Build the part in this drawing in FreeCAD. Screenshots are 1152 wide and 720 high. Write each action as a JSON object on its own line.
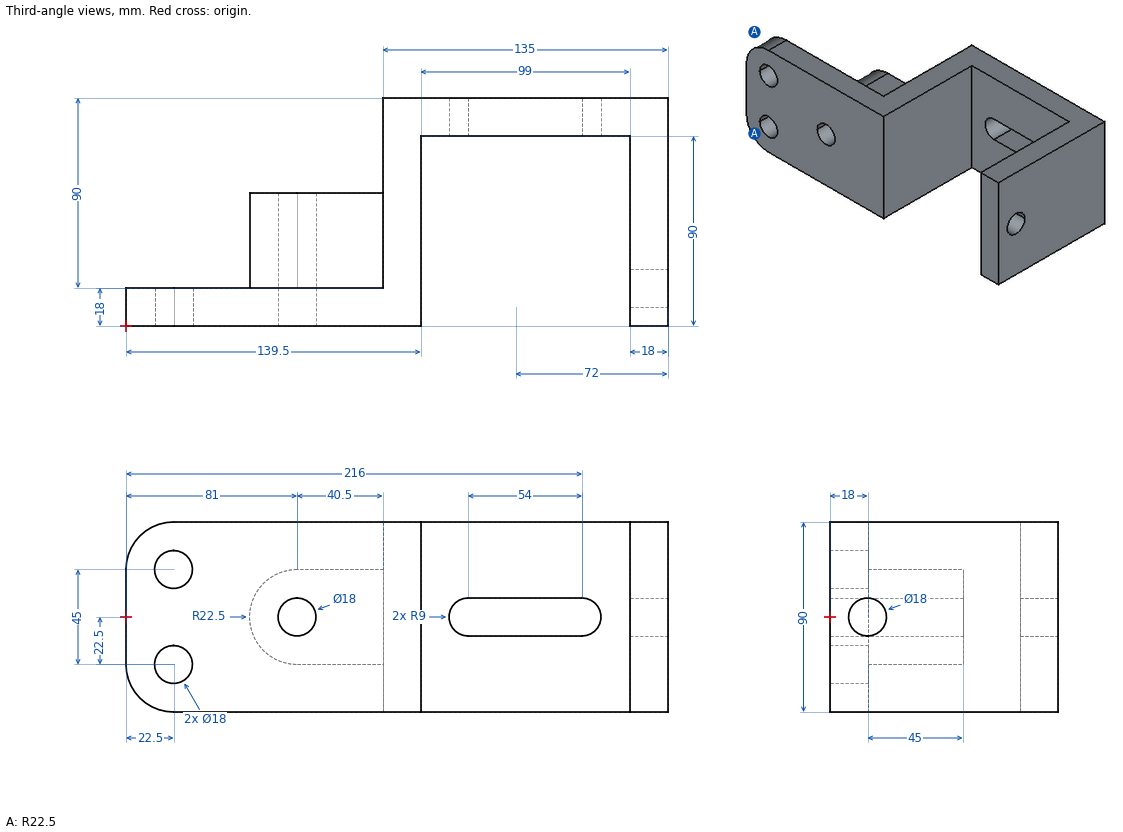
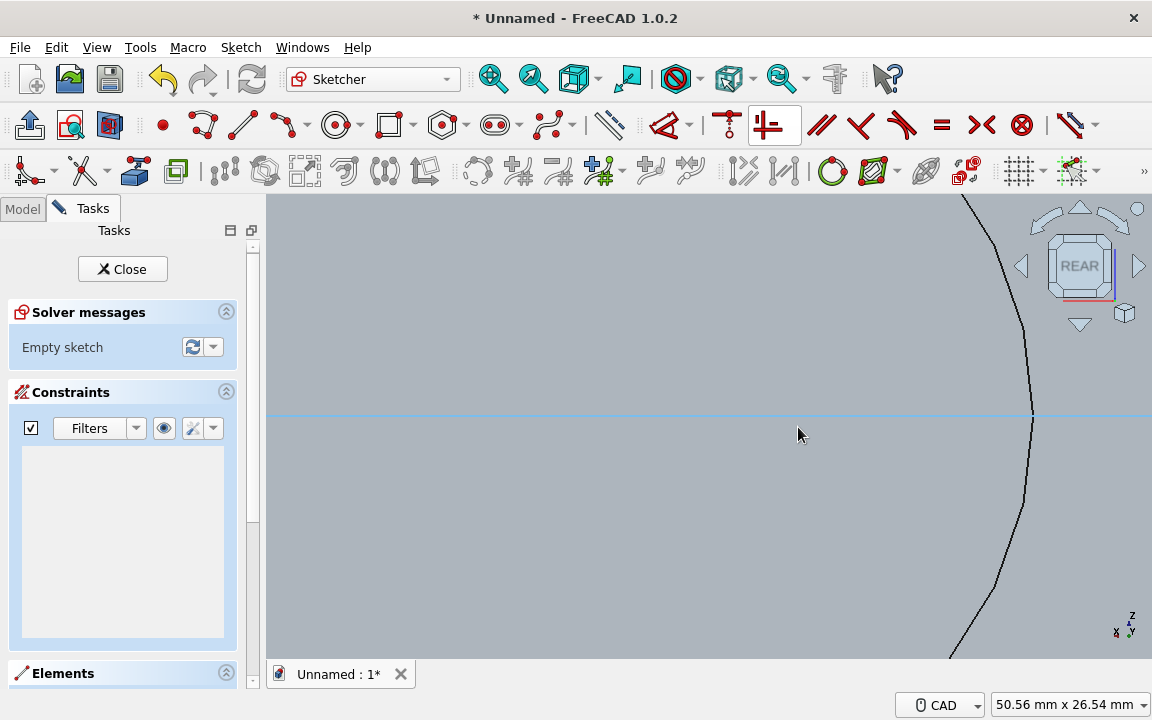
{"action": "left_click", "coordinate": [336, 126]}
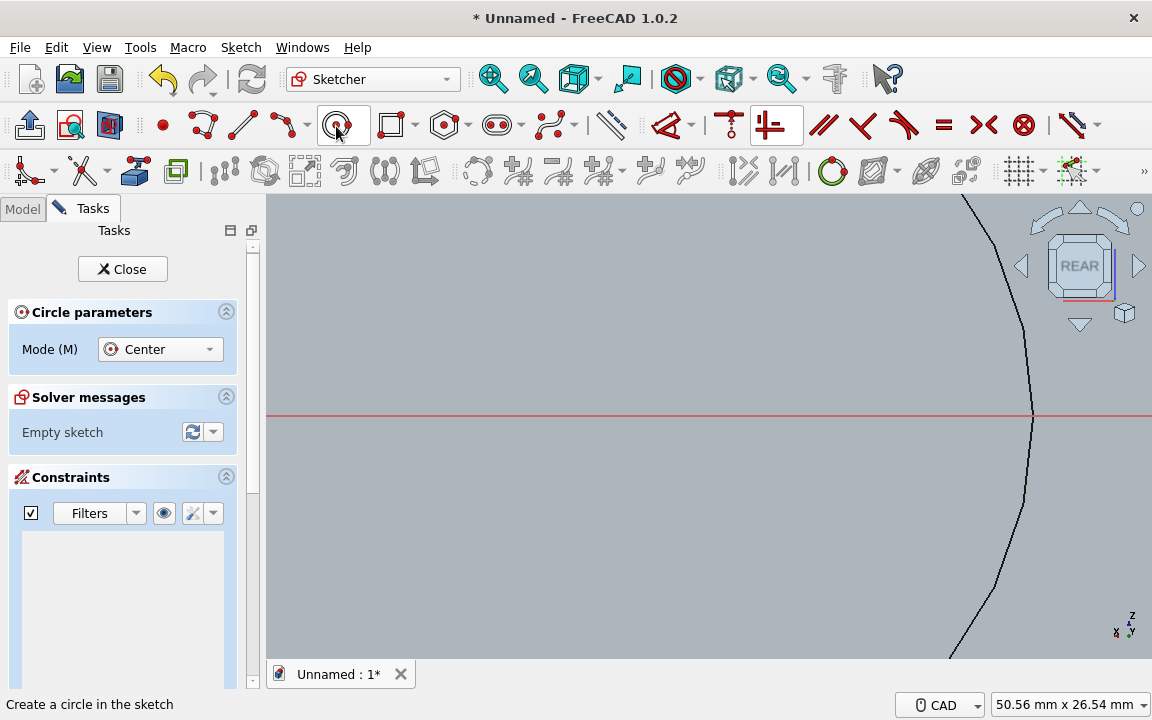
{"action": "left_click", "coordinate": [639, 416]}
{"action": "mouse_move", "coordinate": [750, 305]}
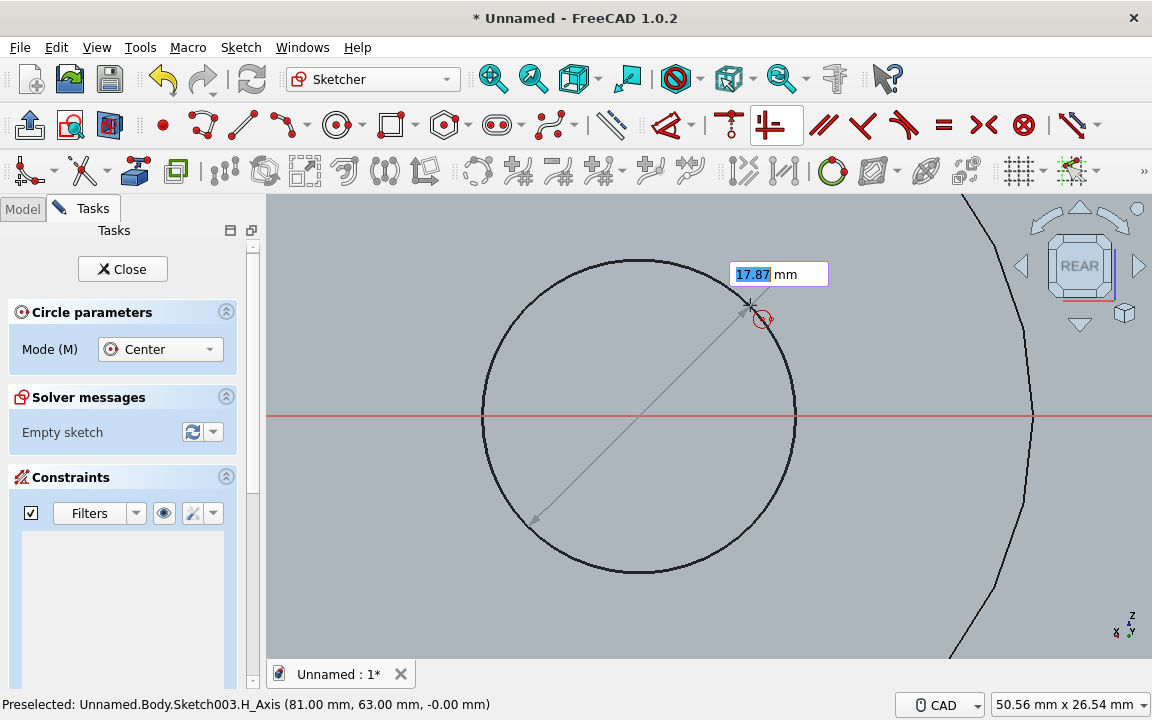
{"action": "type", "text": "18"}
{"action": "key", "text": "Return"}
{"action": "key", "text": "Escape"}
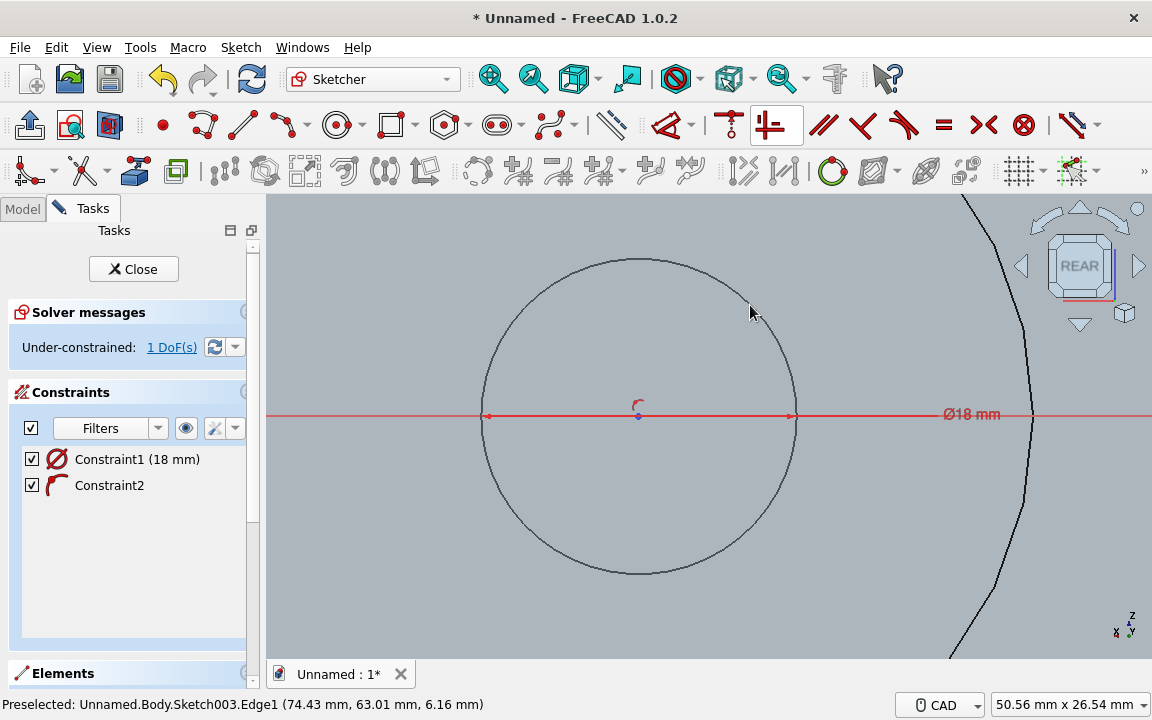
{"action": "left_click", "coordinate": [666, 126]}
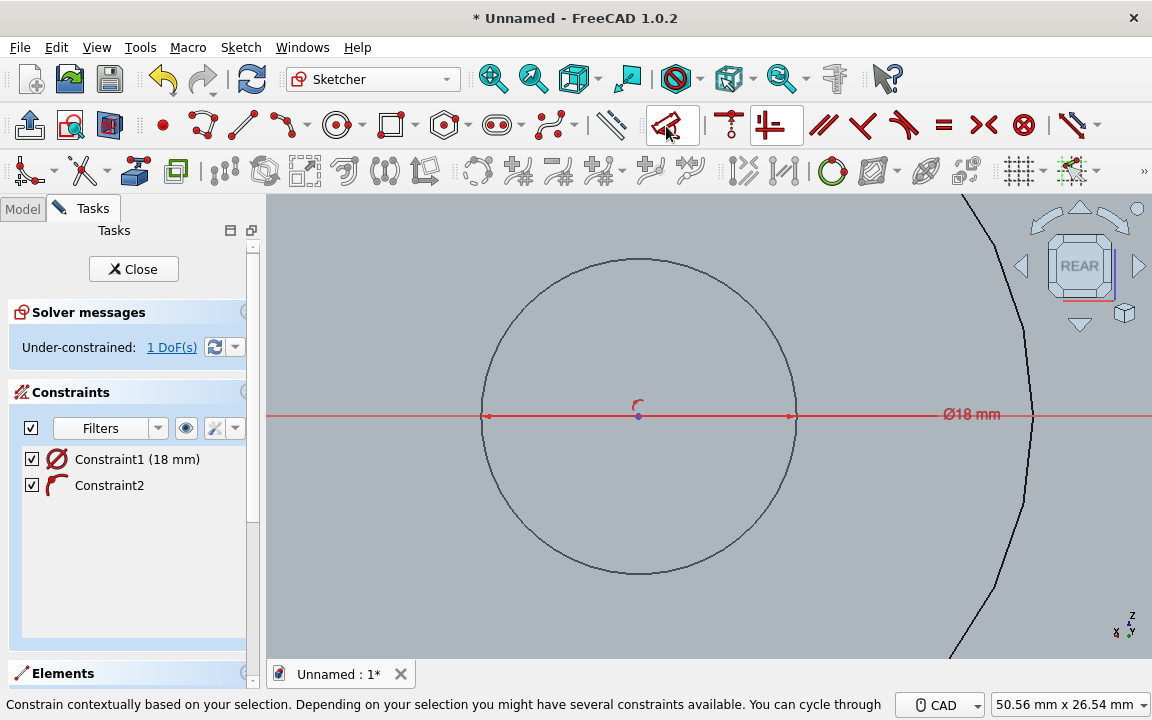
{"action": "left_click", "coordinate": [639, 416]}
{"action": "left_click", "coordinate": [813, 450]}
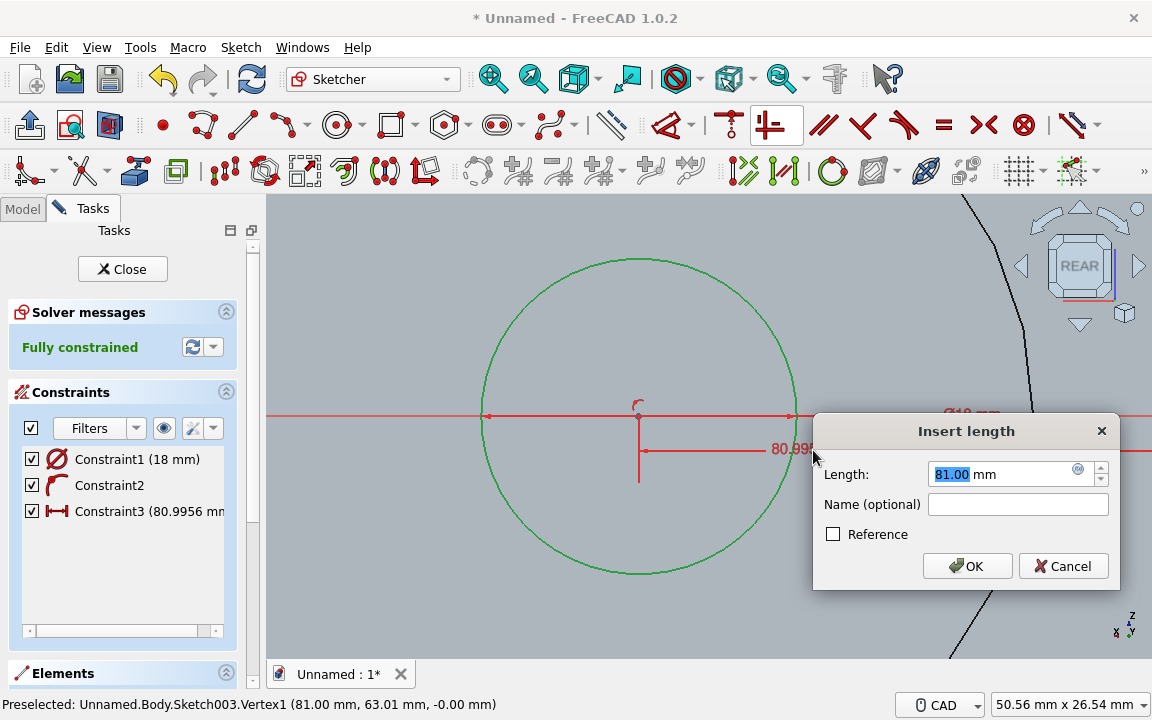
{"action": "type", "text": "81"}
{"action": "key", "text": "Return"}
{"action": "key", "text": "Escape"}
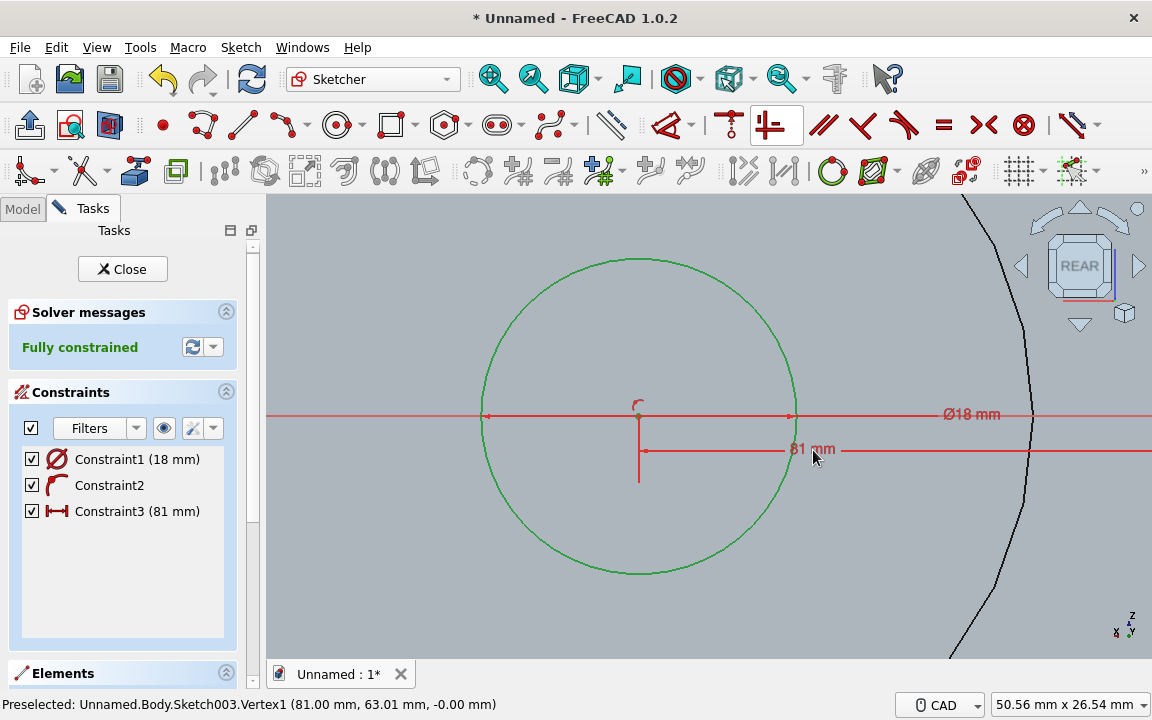
{"action": "left_click", "coordinate": [123, 269]}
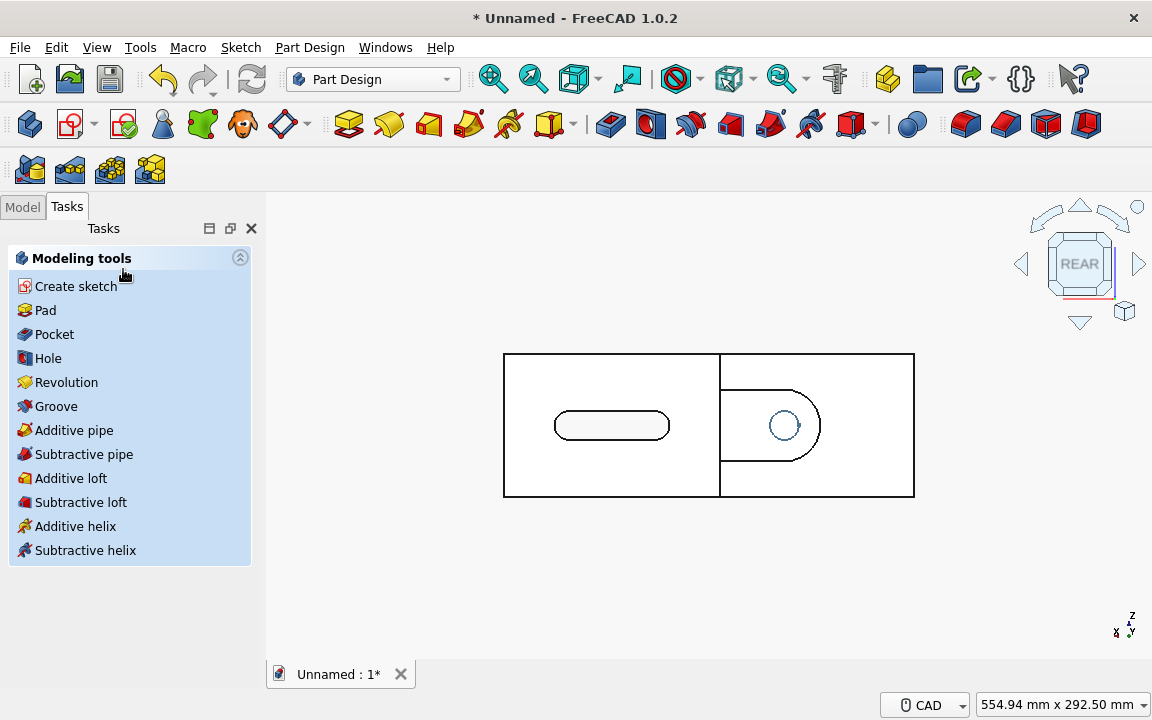
{"action": "left_click", "coordinate": [612, 124]}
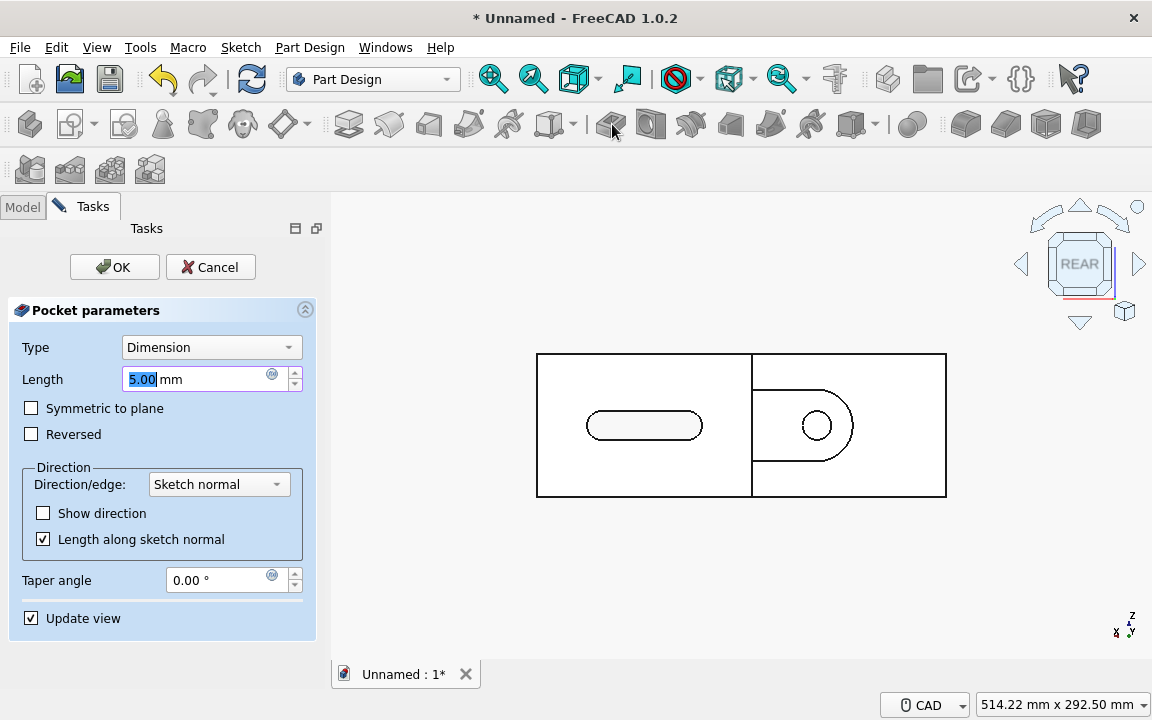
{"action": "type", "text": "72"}
{"action": "key", "text": "Tab"}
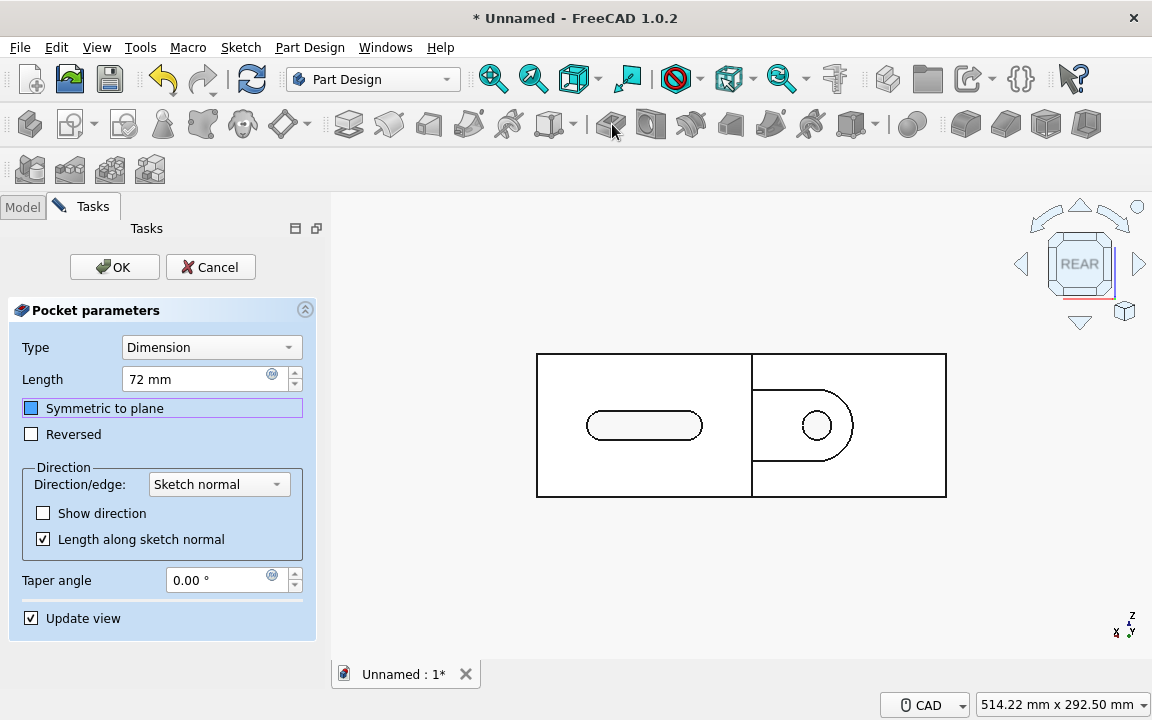
{"action": "left_click", "coordinate": [115, 267]}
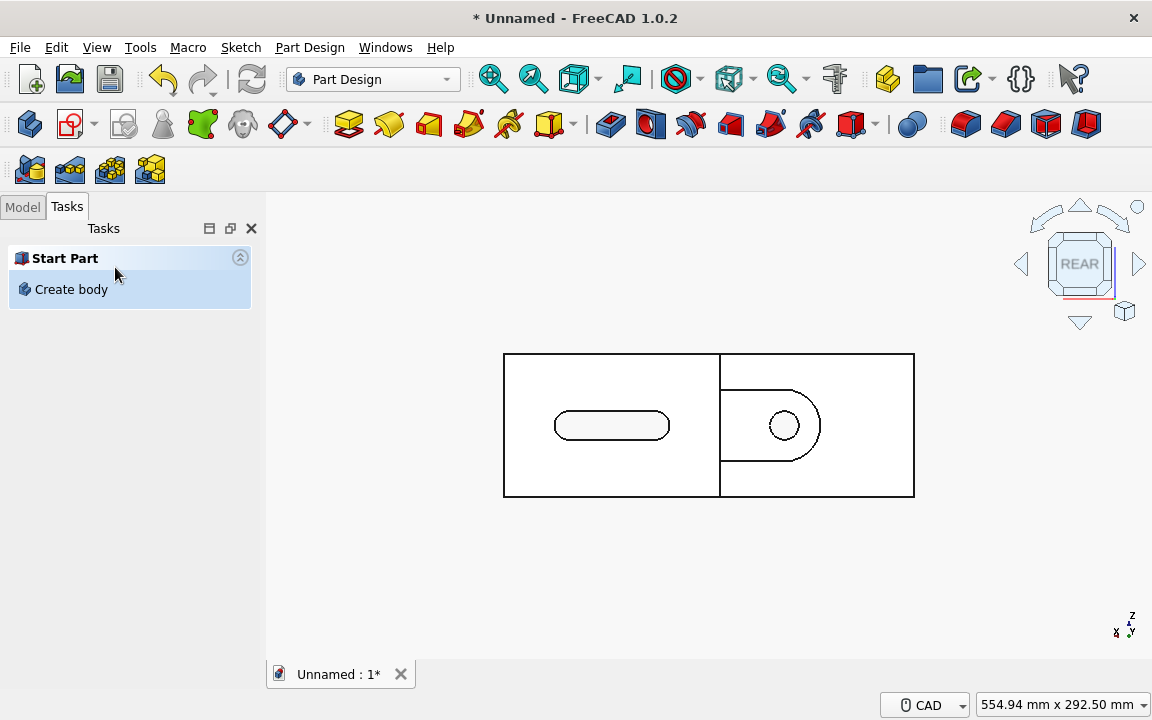
{"action": "key", "text": "0"}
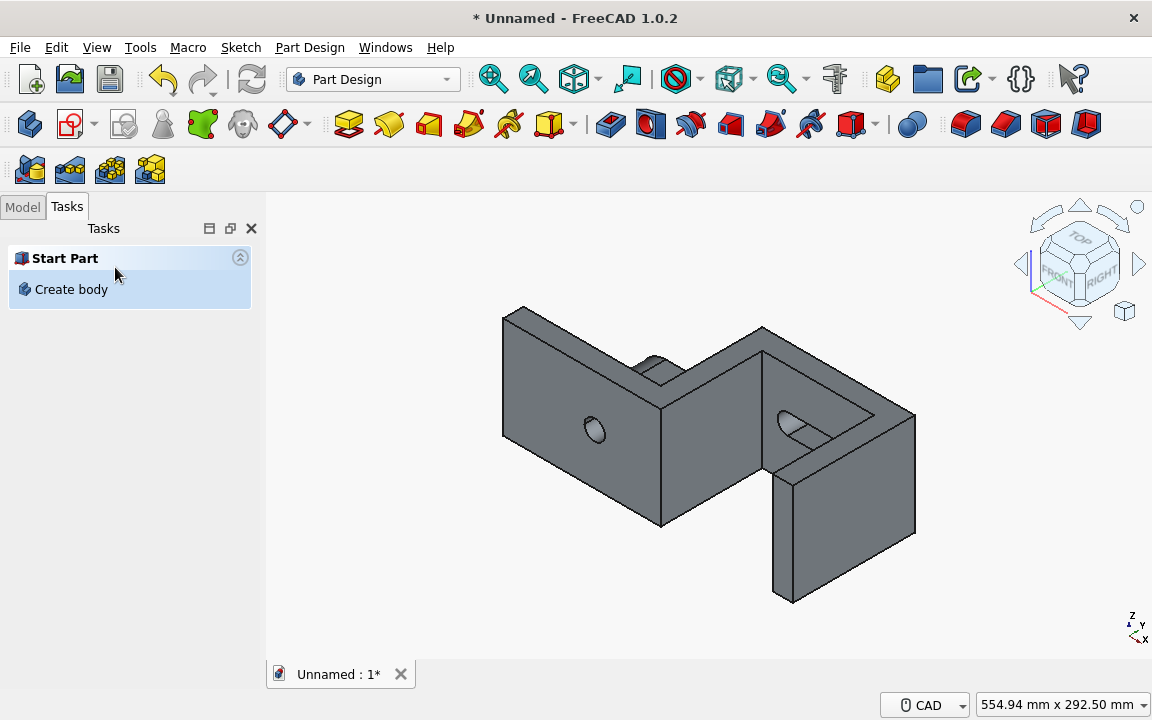
{"action": "key", "text": "2"}